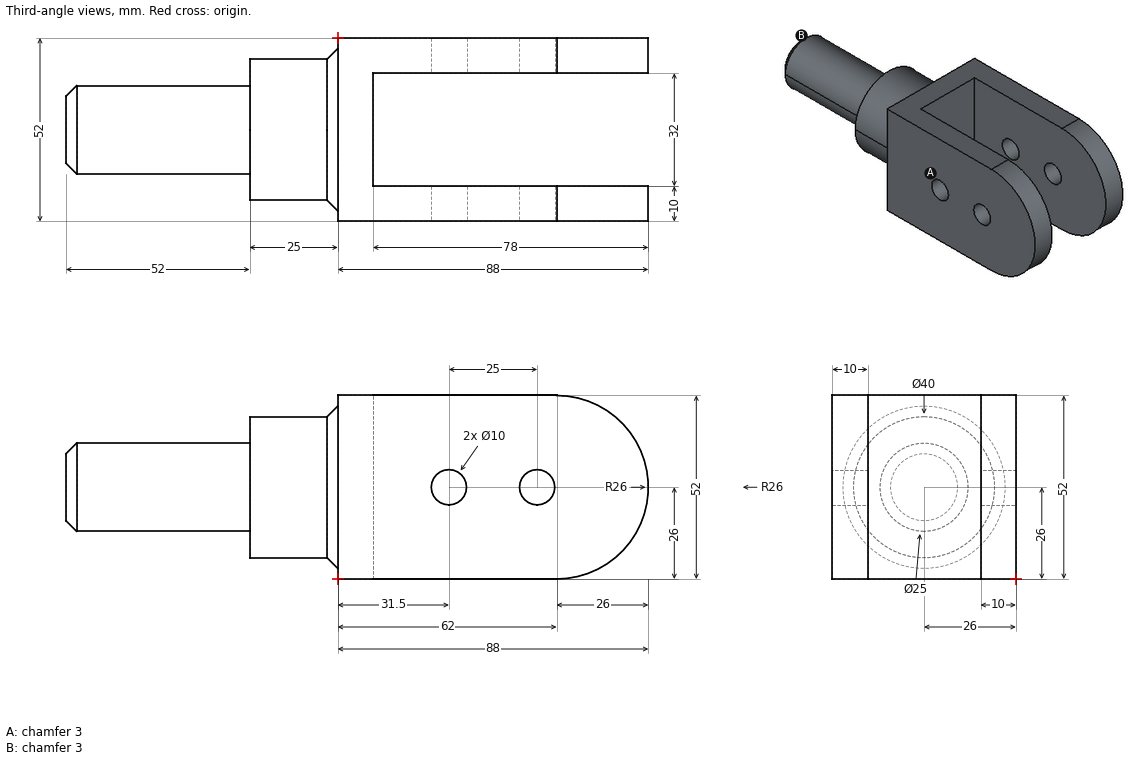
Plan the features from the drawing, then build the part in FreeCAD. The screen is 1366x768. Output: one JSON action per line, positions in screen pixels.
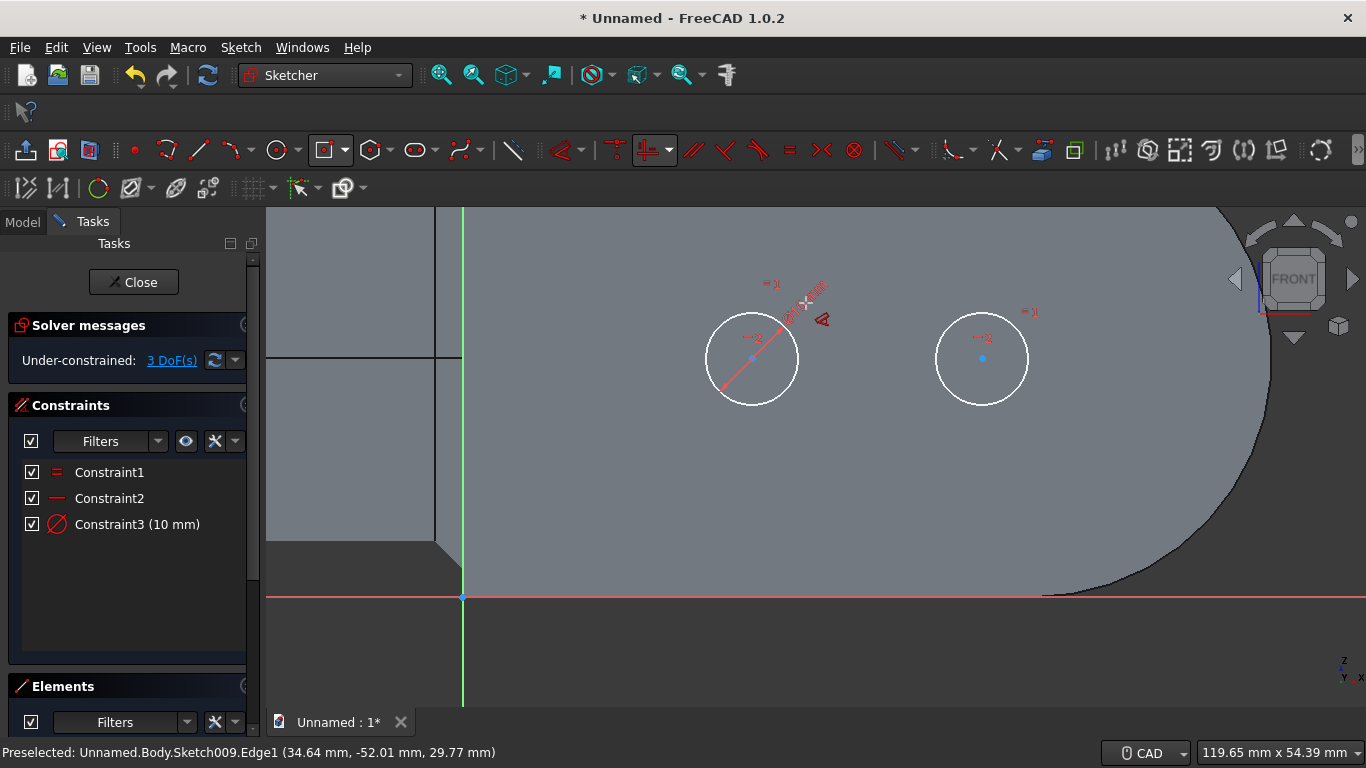
{"action": "left_click", "coordinate": [752, 359]}
{"action": "left_click", "coordinate": [429, 478]}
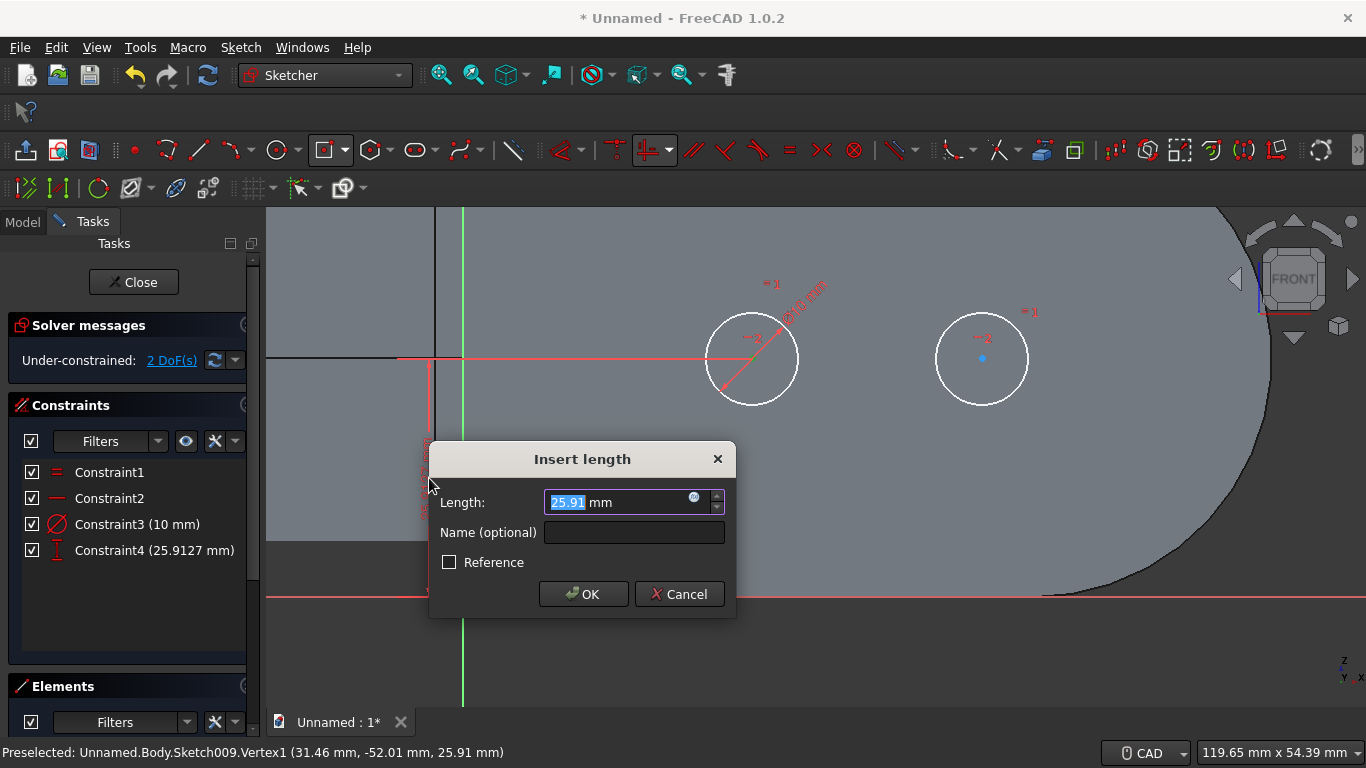
{"action": "type", "text": "26"}
{"action": "key", "text": "Return"}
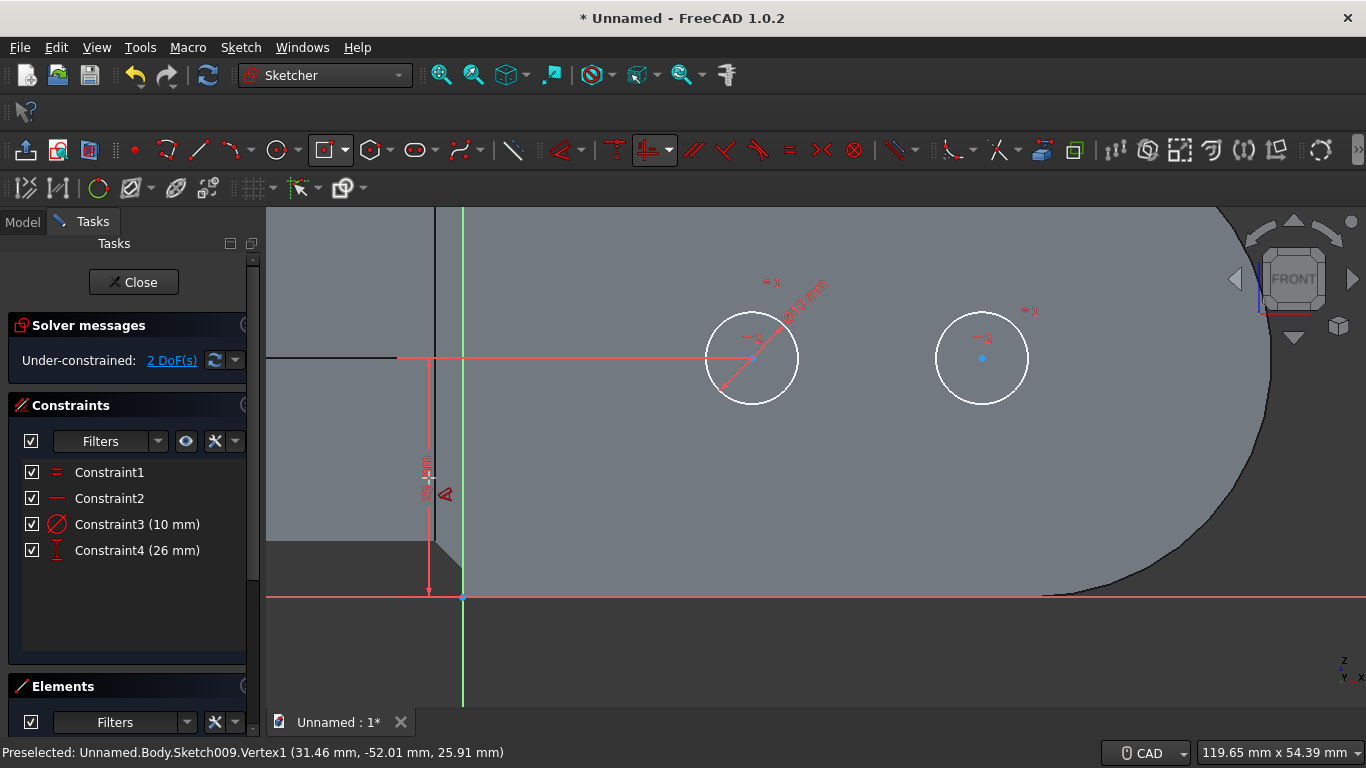
{"action": "left_click", "coordinate": [752, 358]}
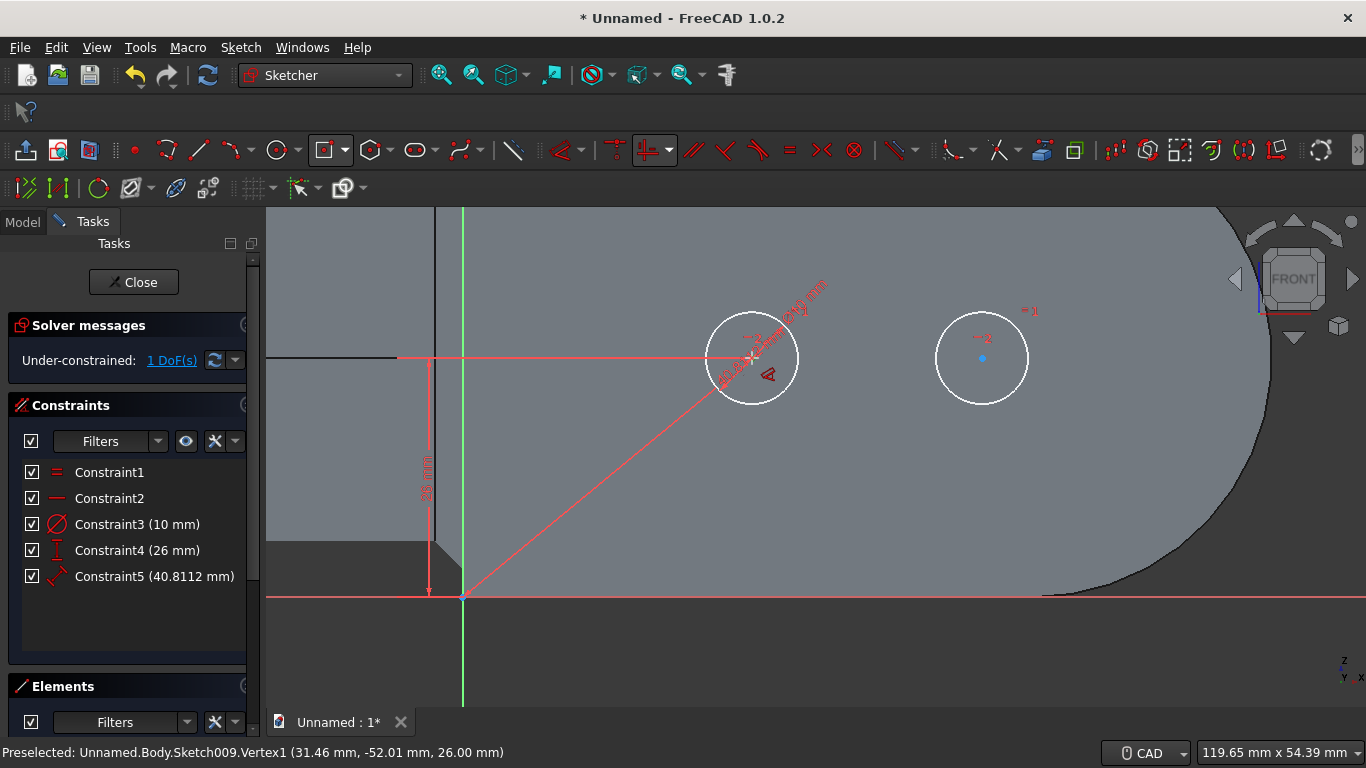
{"action": "left_click", "coordinate": [982, 358]}
{"action": "left_click", "coordinate": [867, 324]}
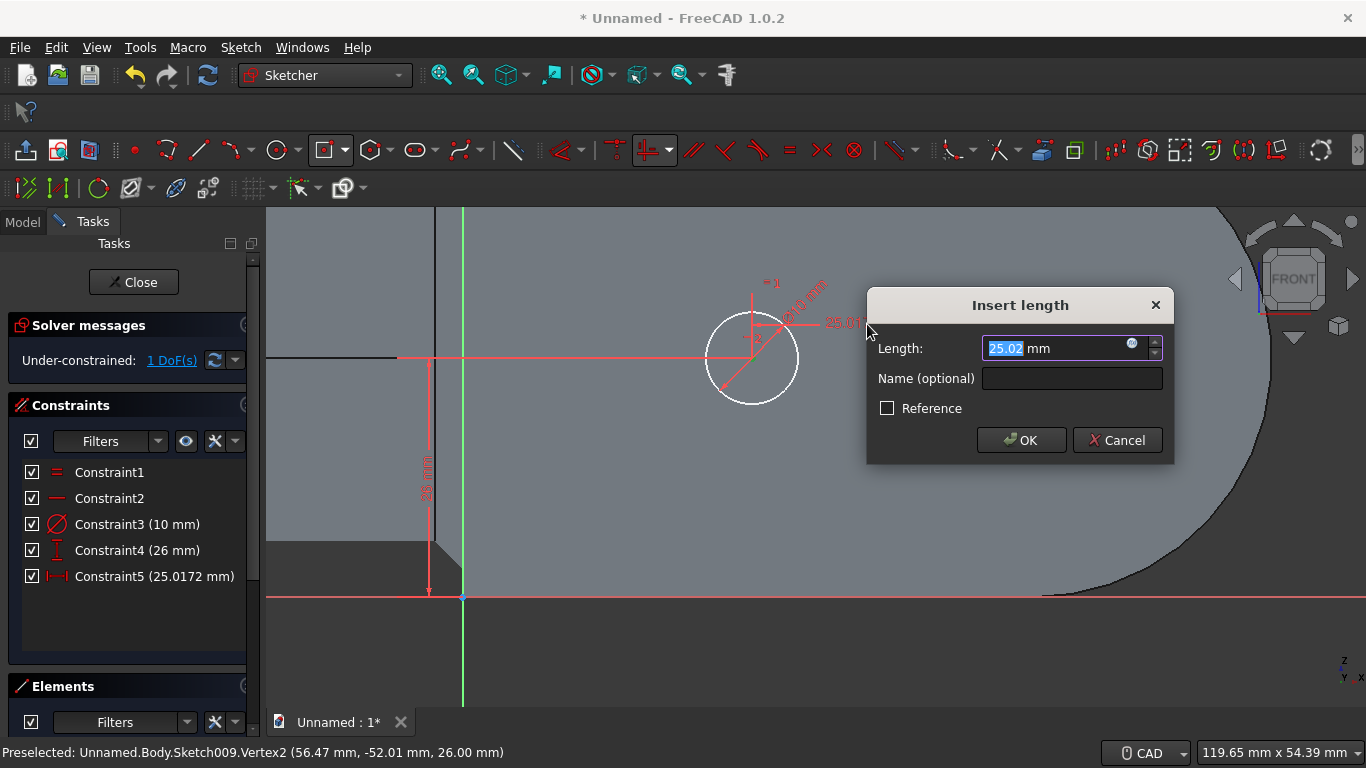
{"action": "type", "text": "25"}
{"action": "key", "text": "Return"}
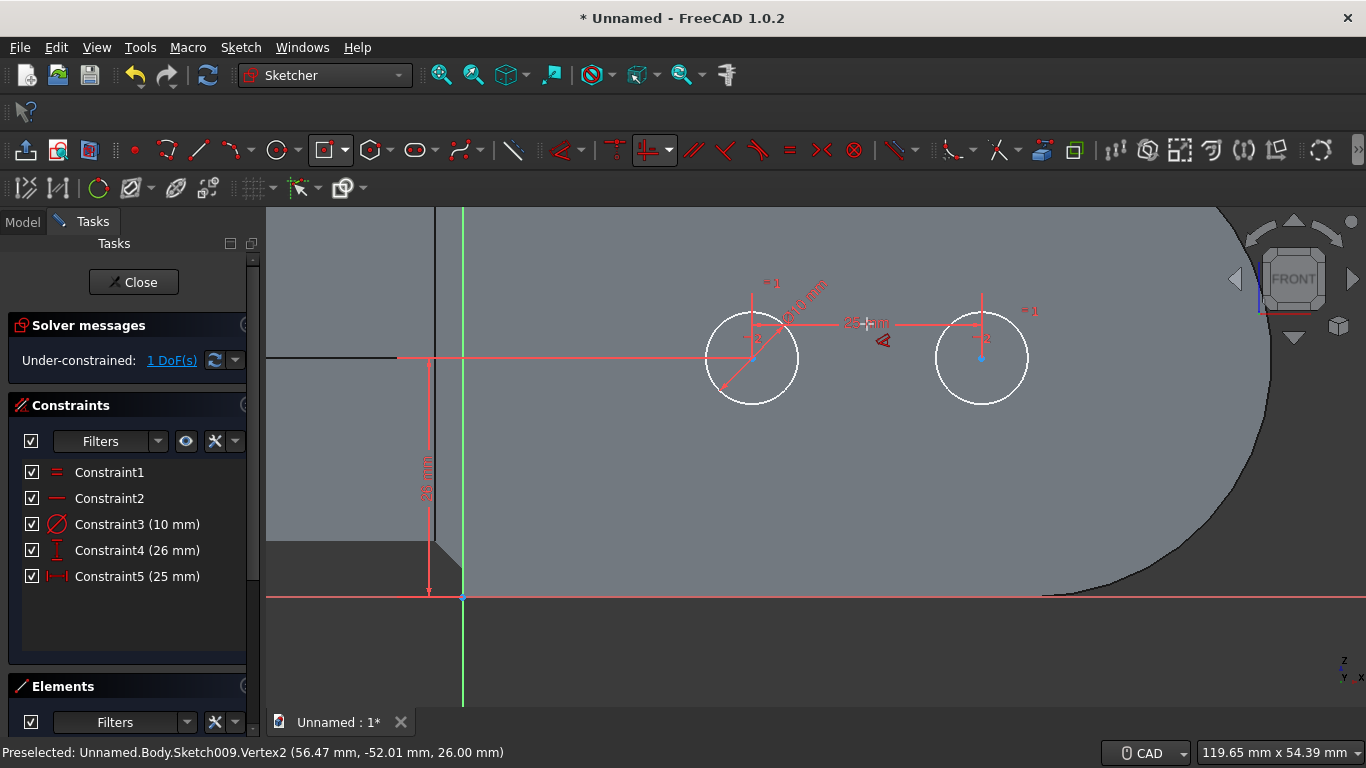
{"action": "left_click", "coordinate": [752, 358]}
{"action": "left_click", "coordinate": [607, 631]}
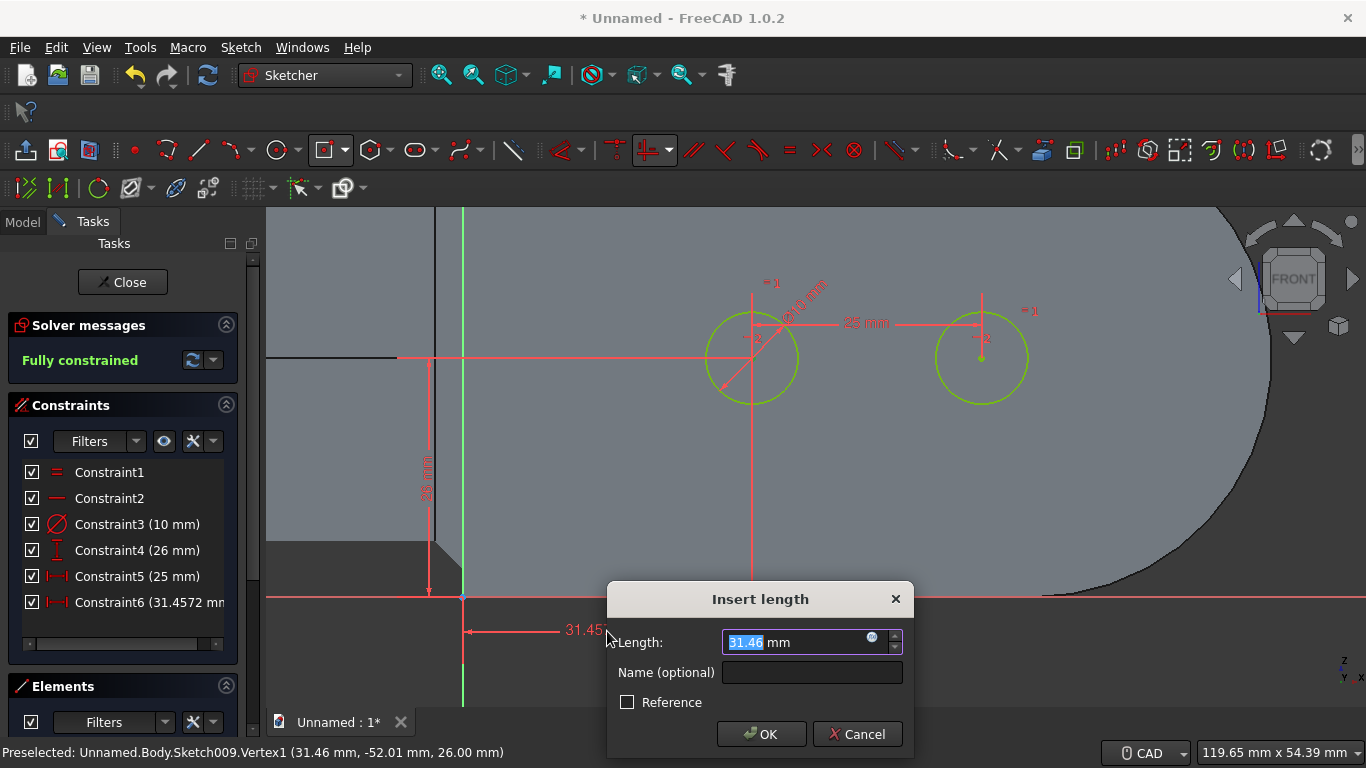
{"action": "type", "text": "31.5"}
{"action": "key", "text": "Return"}
{"action": "key", "text": "Escape"}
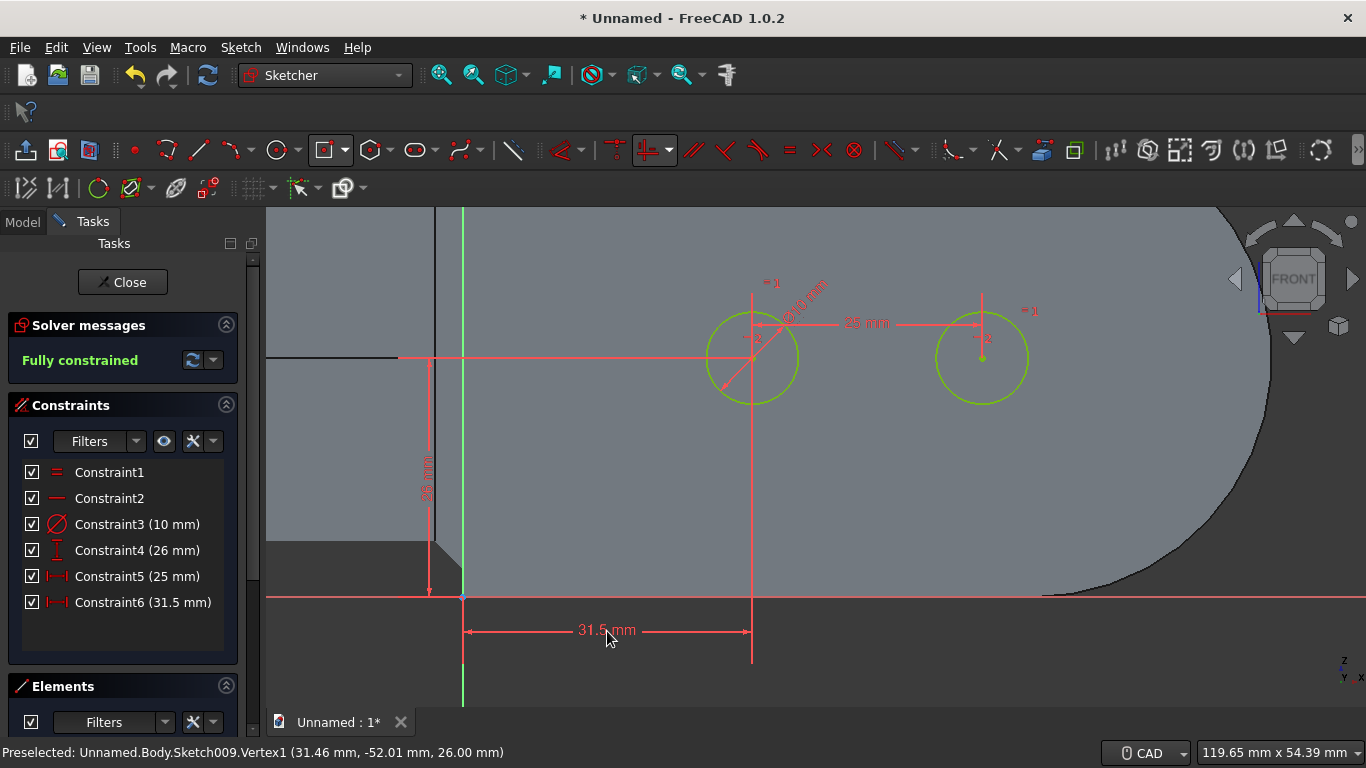
{"action": "left_click", "coordinate": [123, 282]}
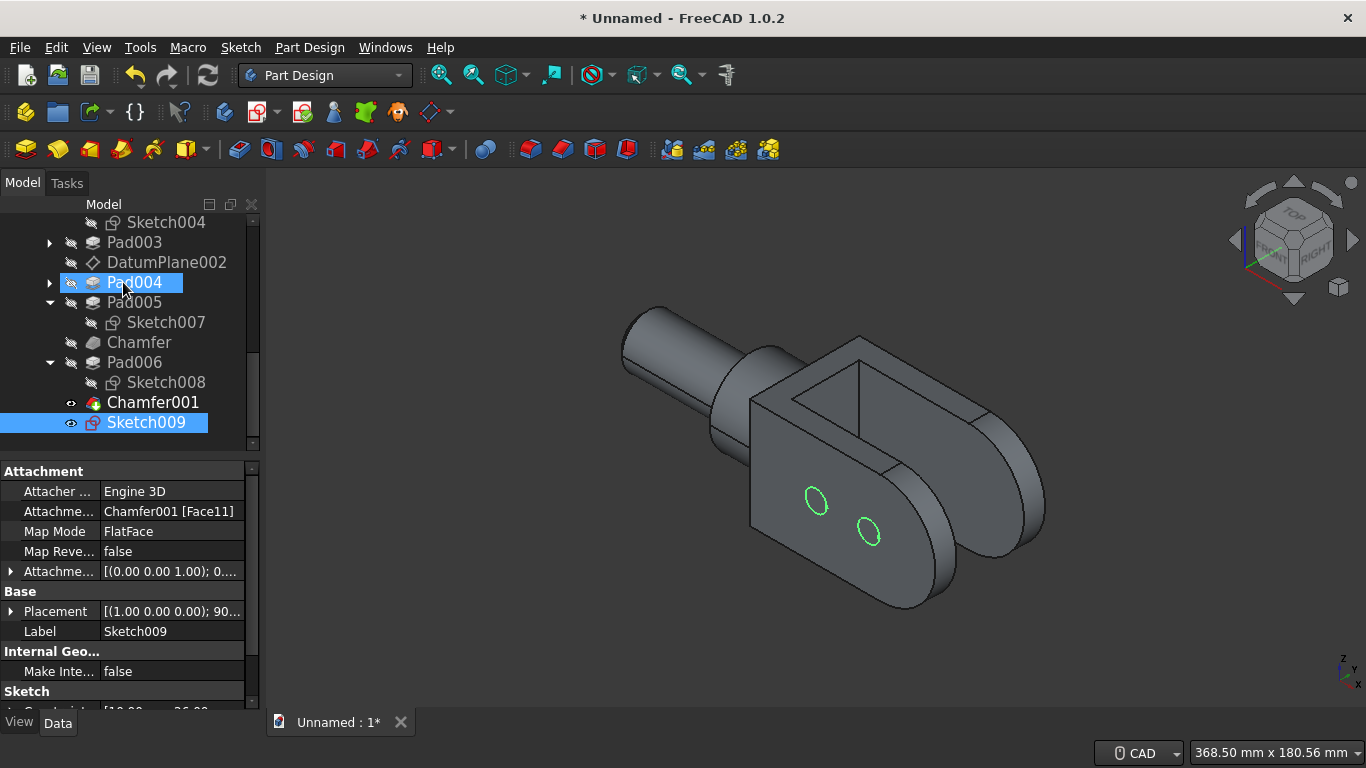
{"action": "left_click", "coordinate": [240, 150]}